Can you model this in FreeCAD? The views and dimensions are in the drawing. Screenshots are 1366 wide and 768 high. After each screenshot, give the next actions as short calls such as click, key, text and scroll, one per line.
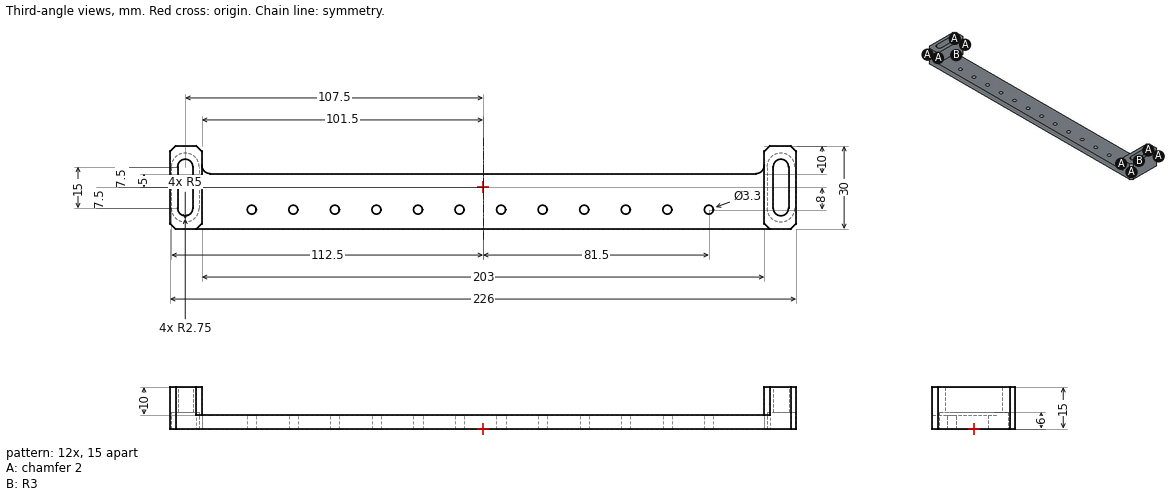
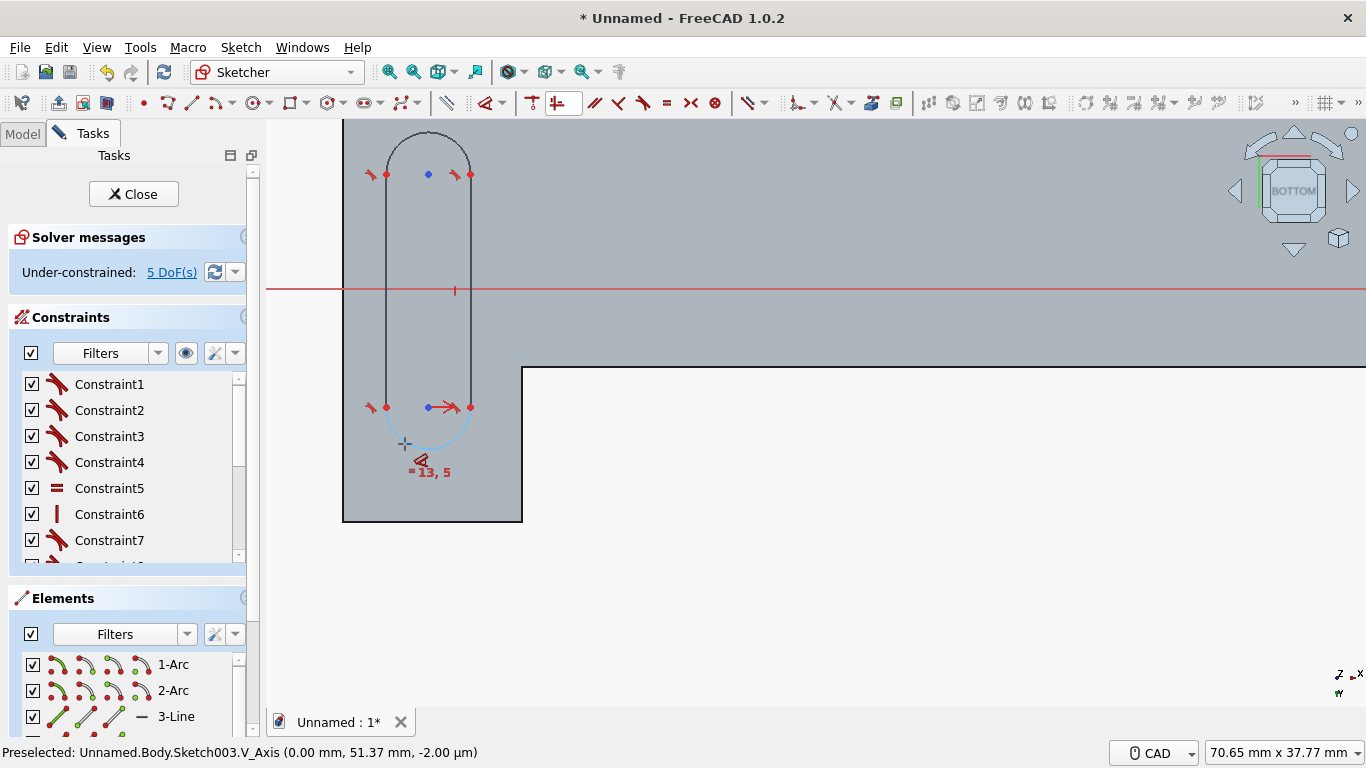
click(404, 441)
click(385, 467)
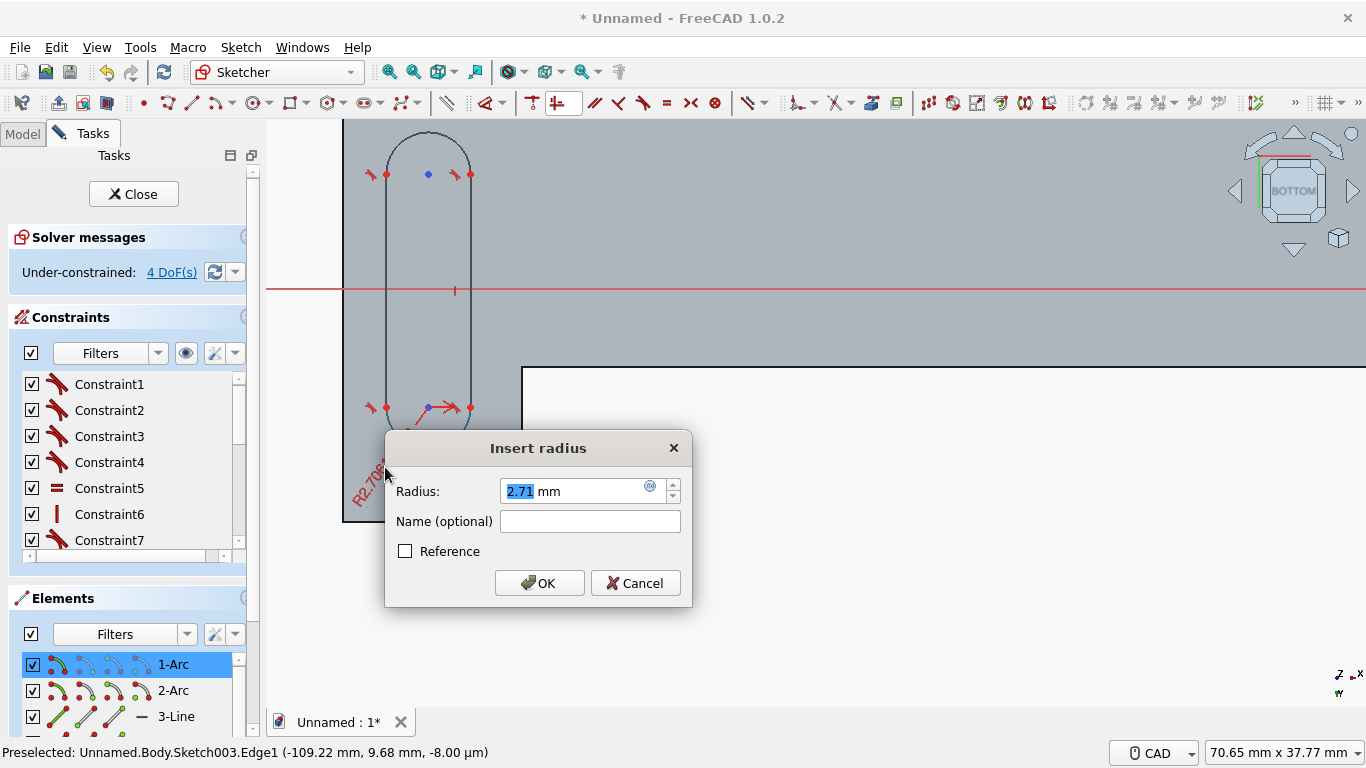
text(2.75)
key(Return)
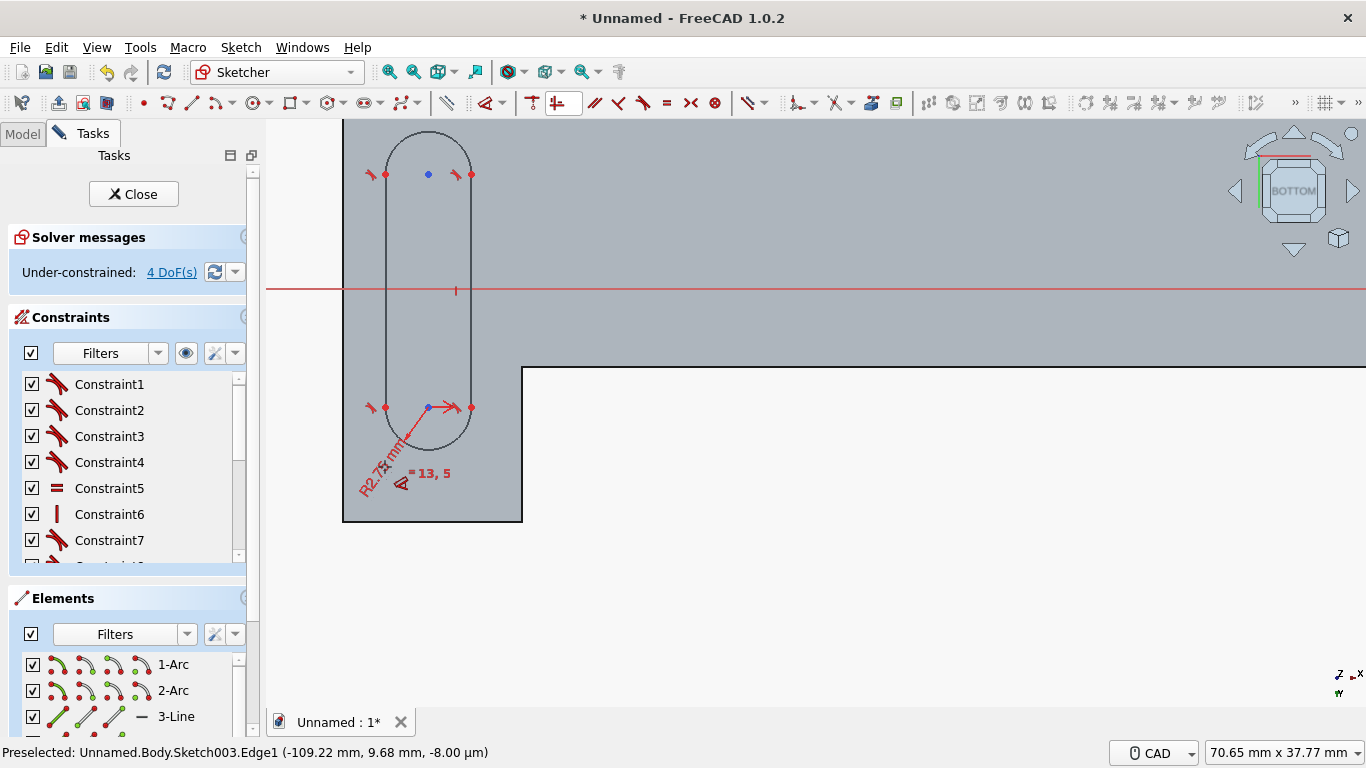
scroll(405, 444, down, 8)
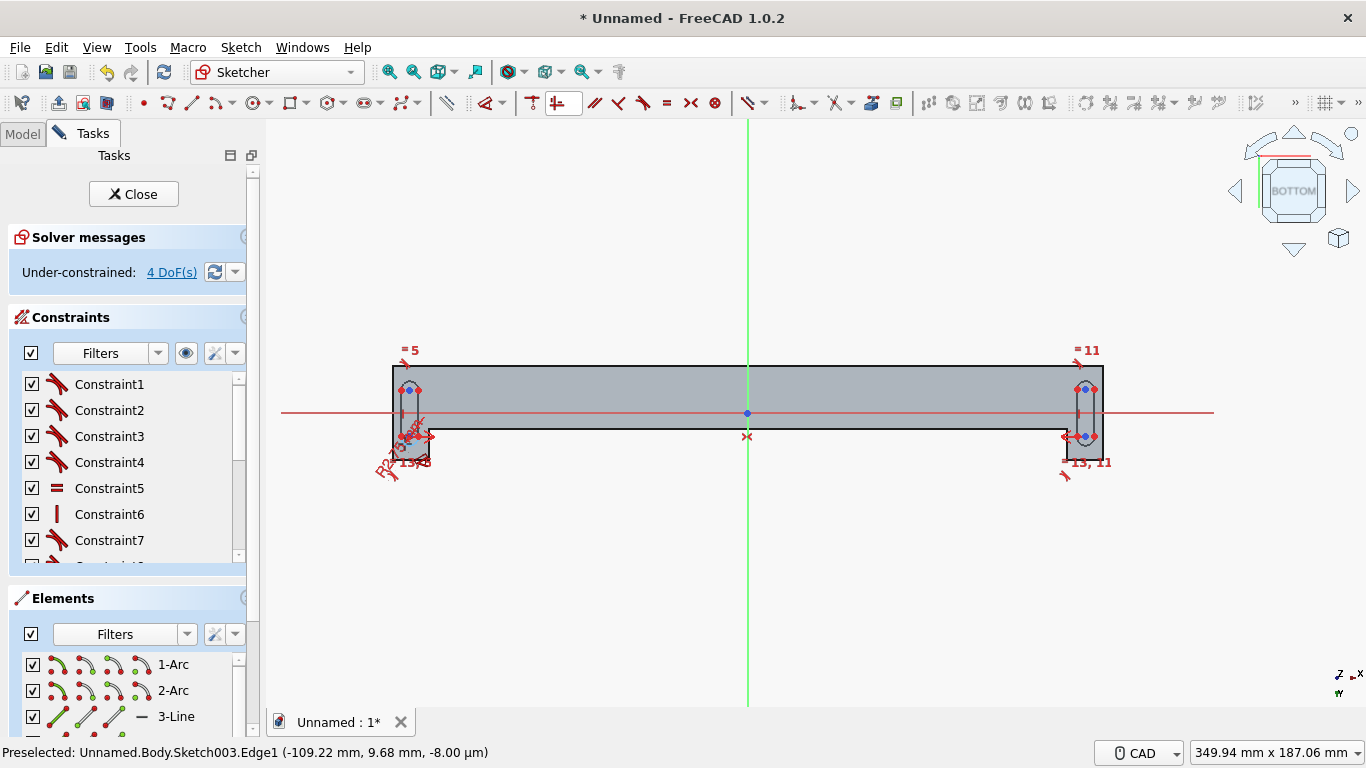
scroll(401, 423, up, 2)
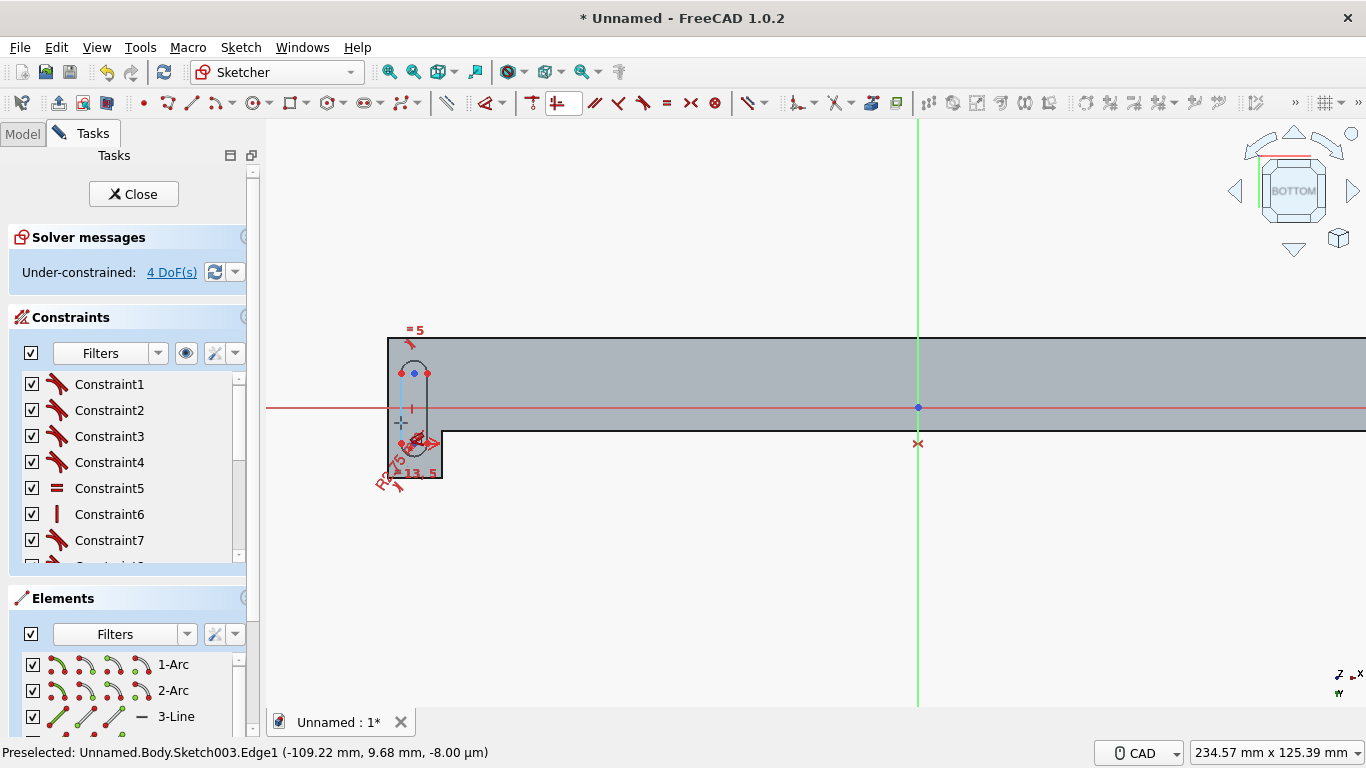
click(401, 423)
click(367, 392)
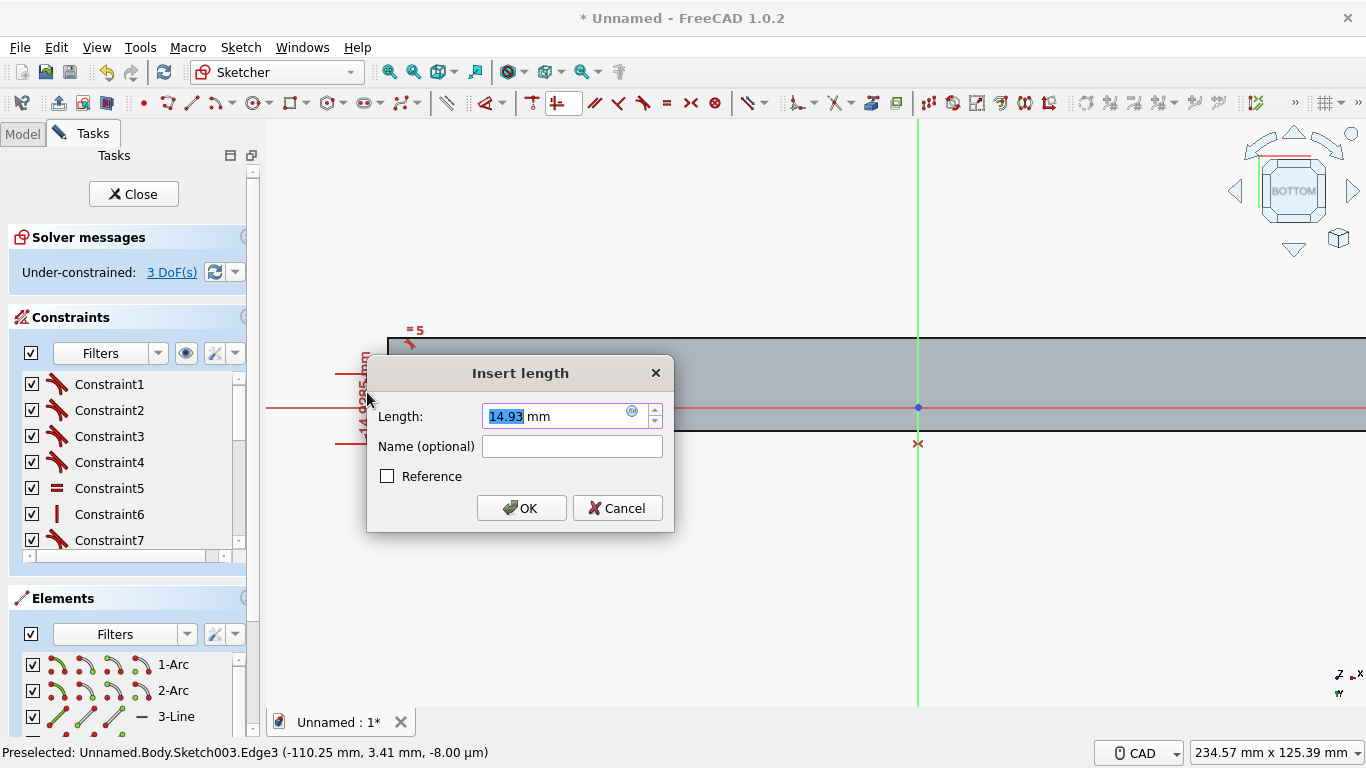
text(15)
key(Return)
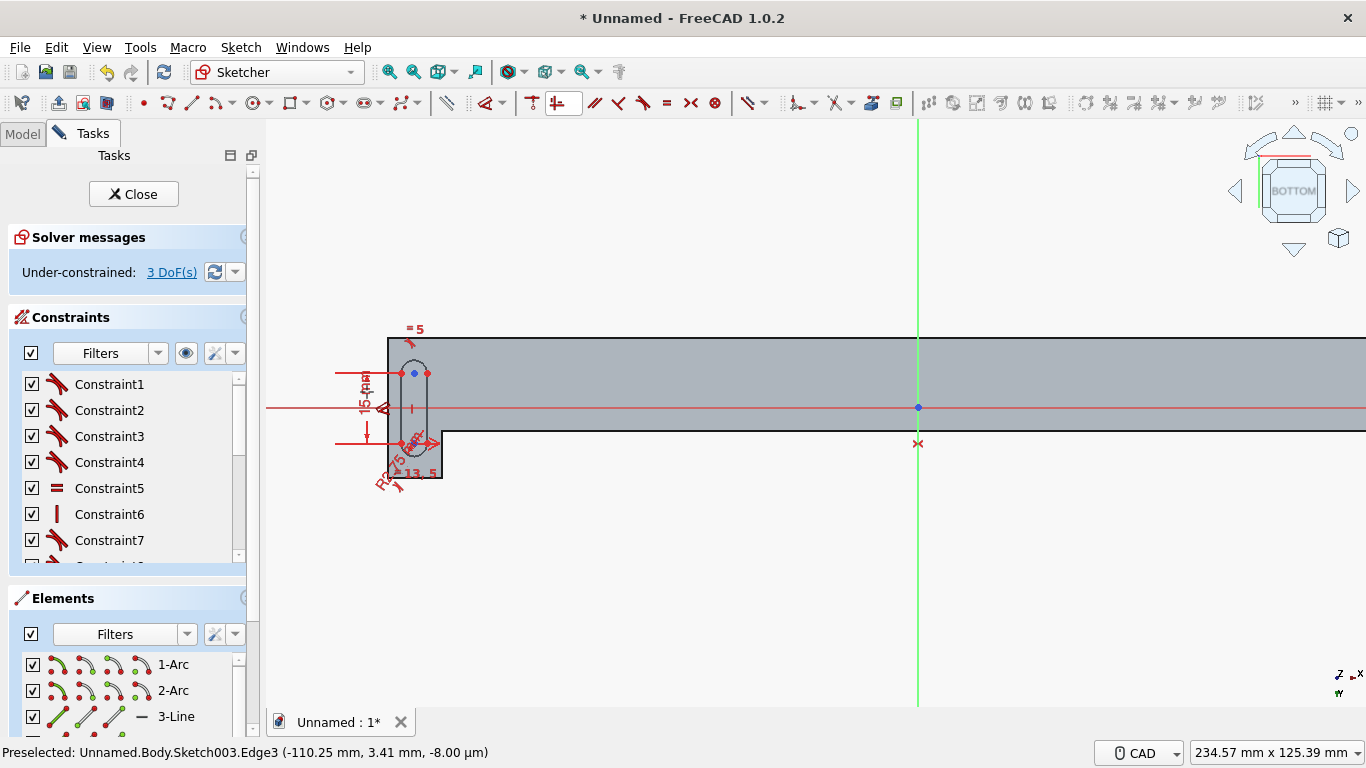
scroll(400, 423, down, 2)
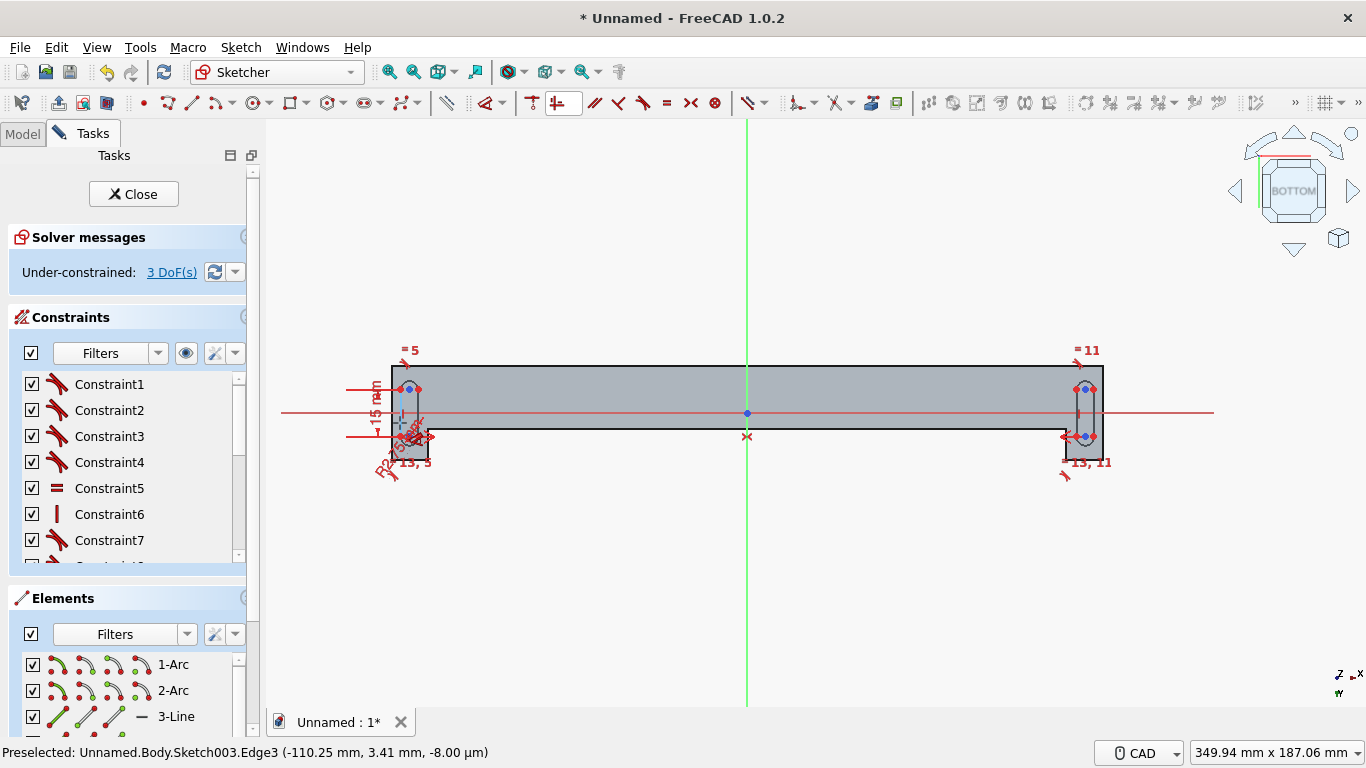
scroll(1077, 423, up, 2)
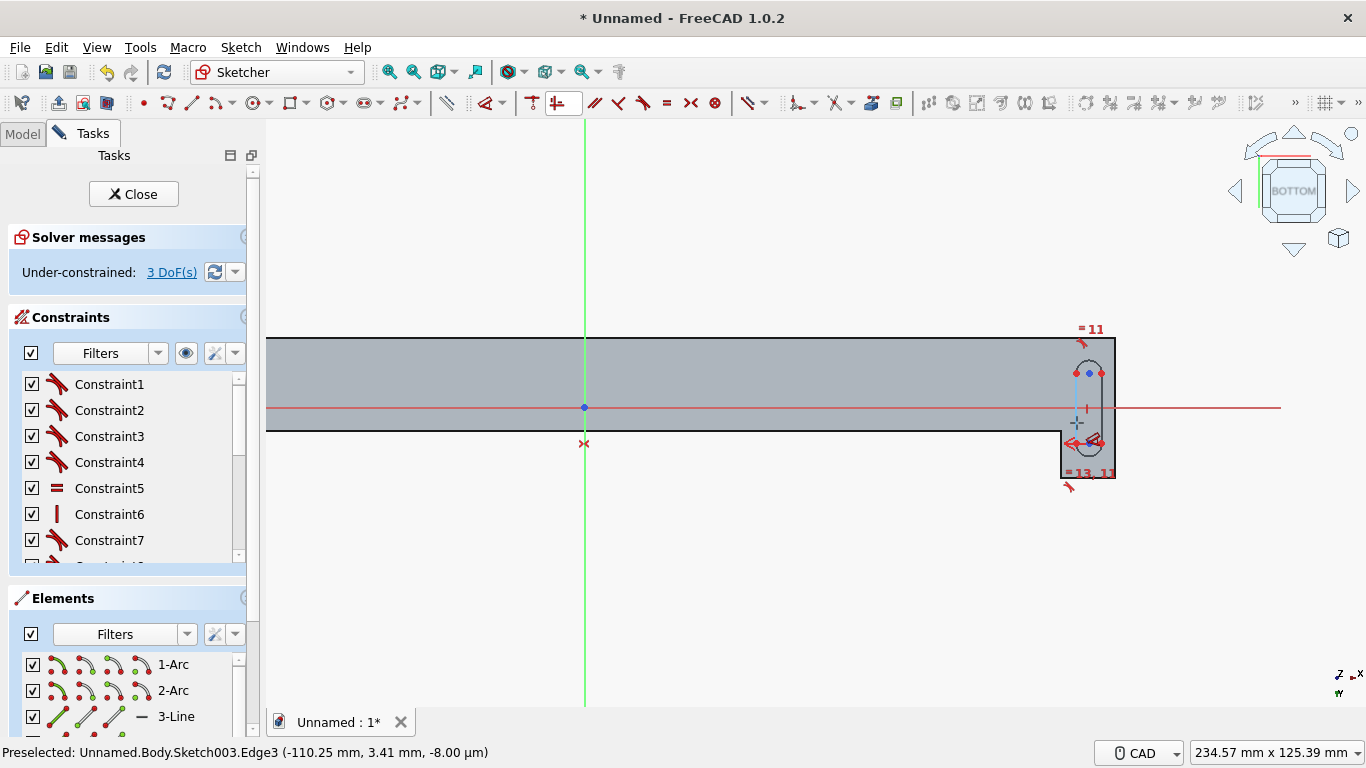
click(1076, 423)
click(1042, 392)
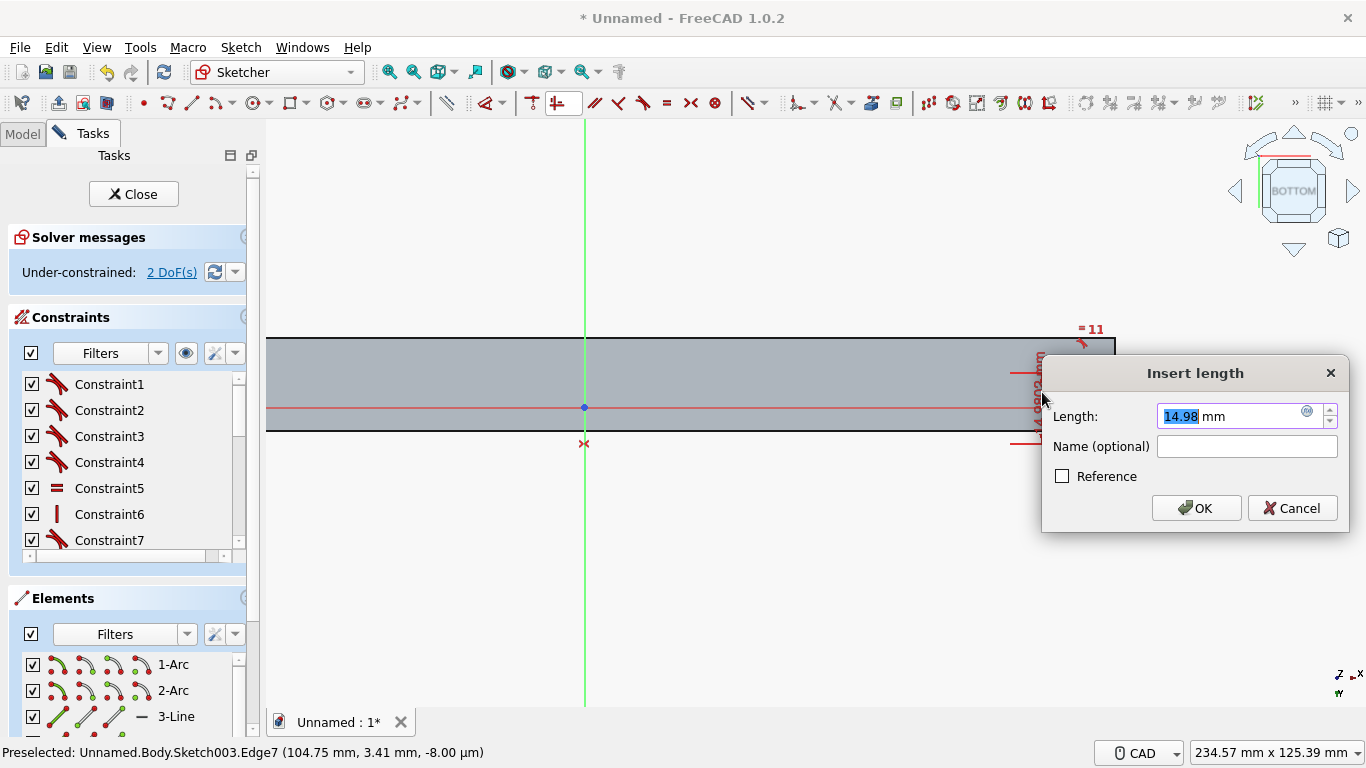
text(15)
key(Return)